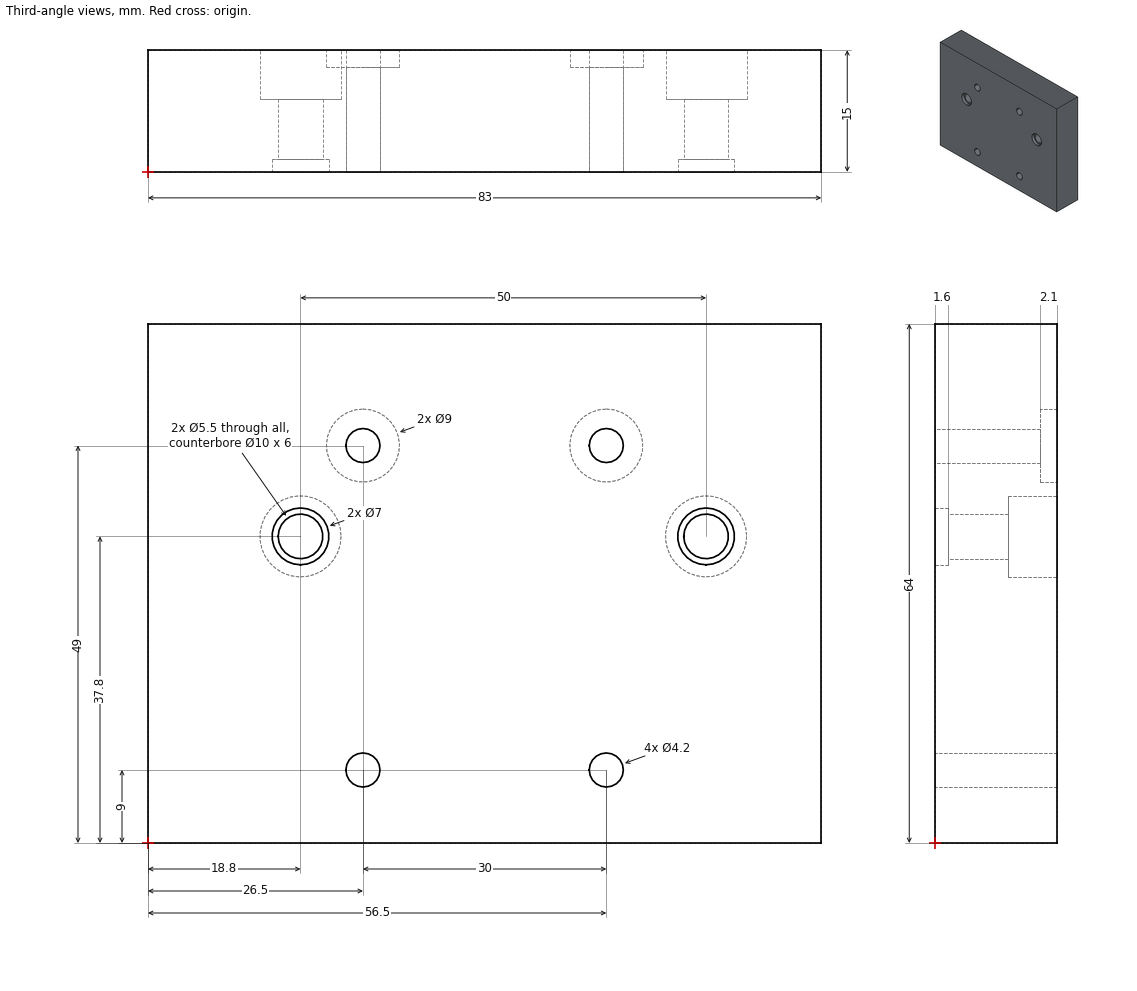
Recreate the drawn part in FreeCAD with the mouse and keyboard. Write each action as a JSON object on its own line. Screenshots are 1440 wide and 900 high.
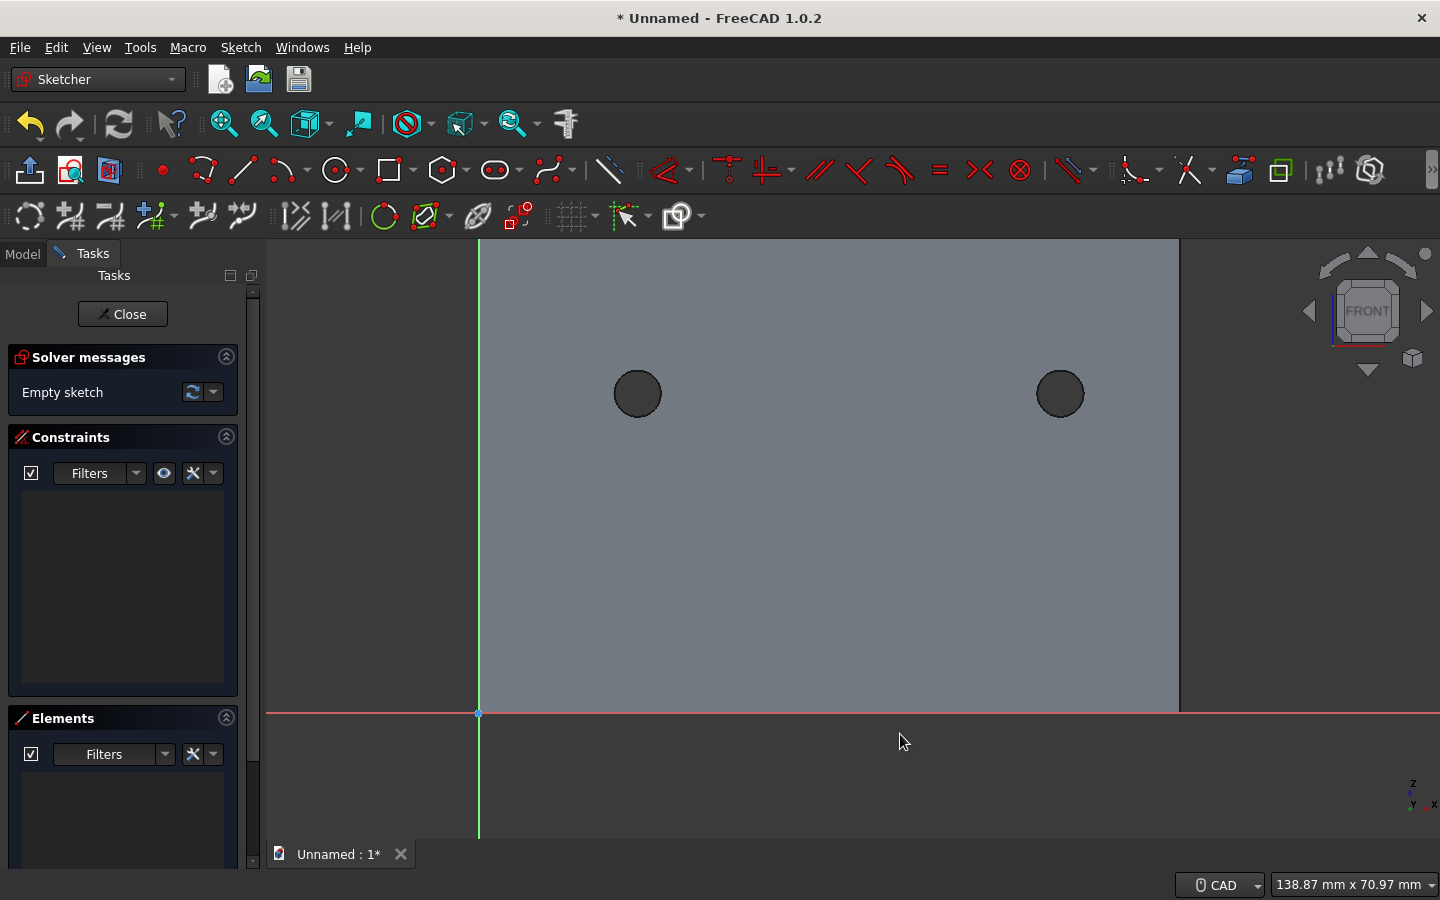
{"action": "left_click", "coordinate": [336, 170]}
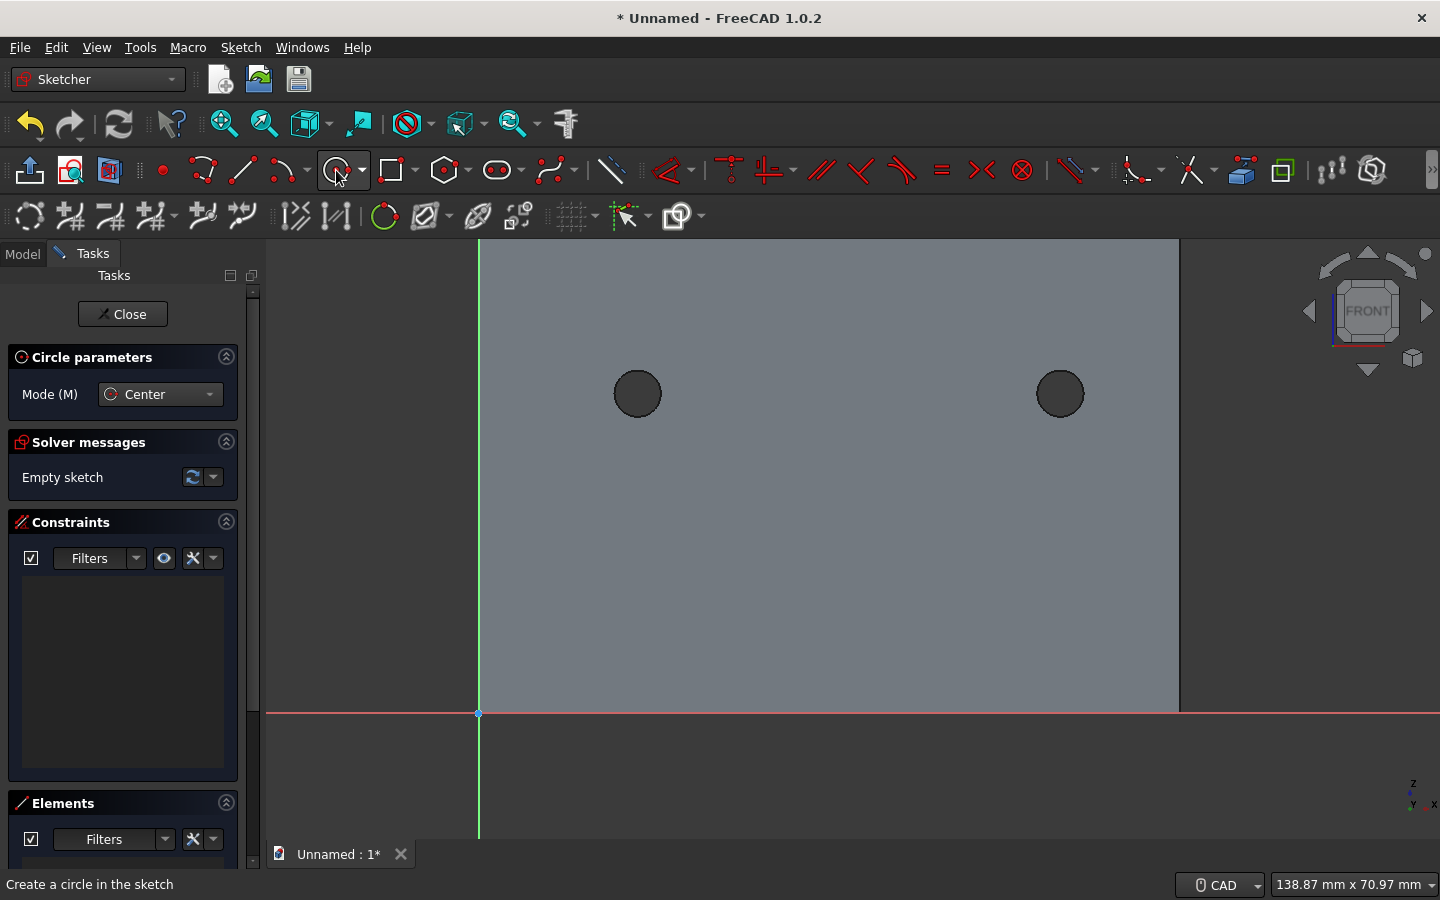
{"action": "left_click", "coordinate": [638, 394]}
{"action": "left_click", "coordinate": [659, 373]}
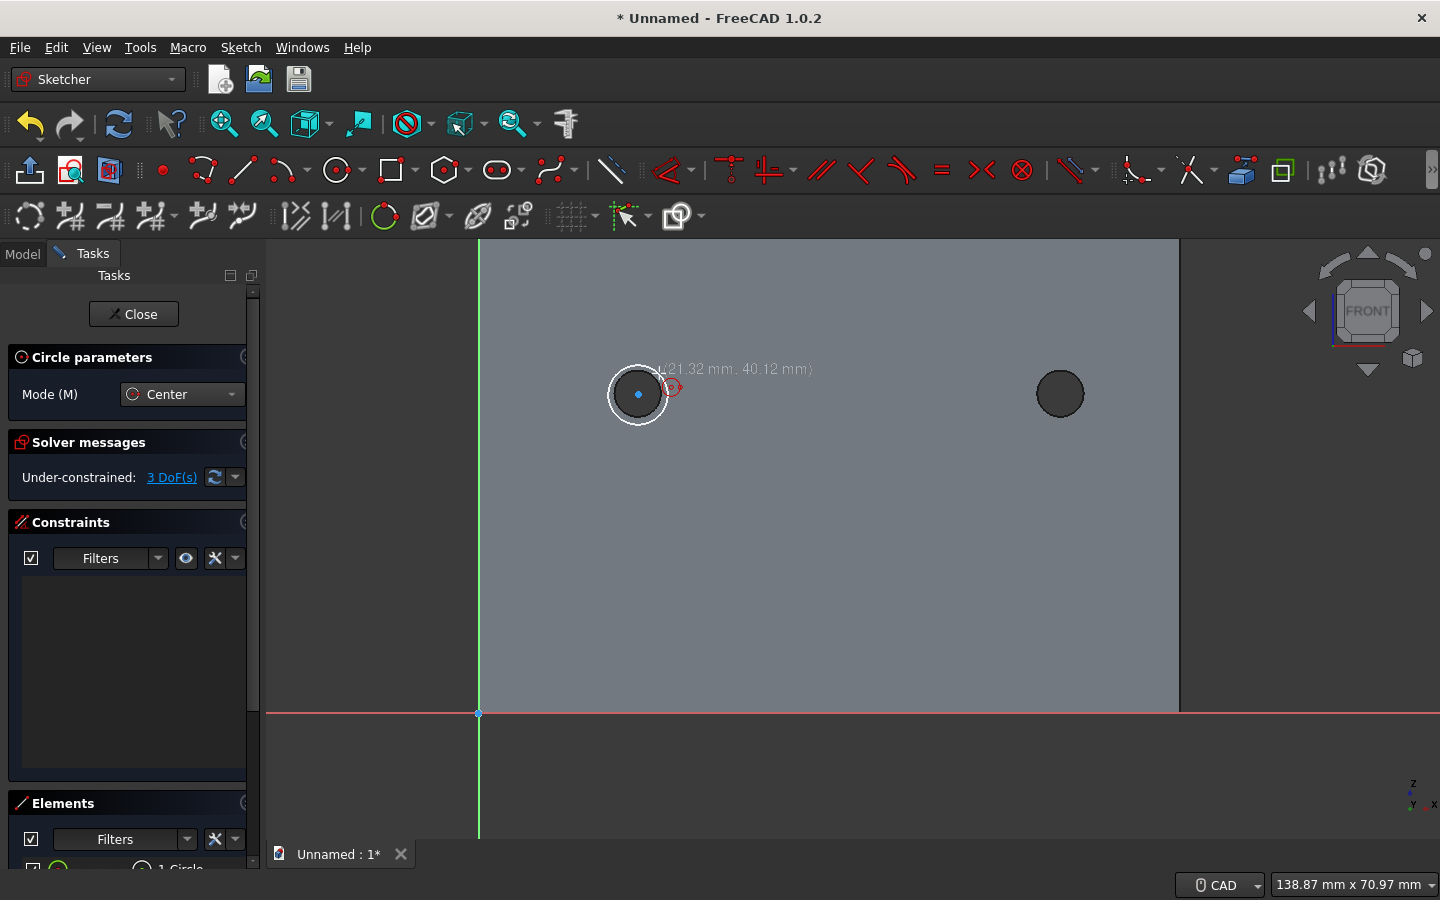
{"action": "left_click", "coordinate": [1060, 394]}
{"action": "left_click", "coordinate": [1081, 373]}
{"action": "key", "text": "Escape"}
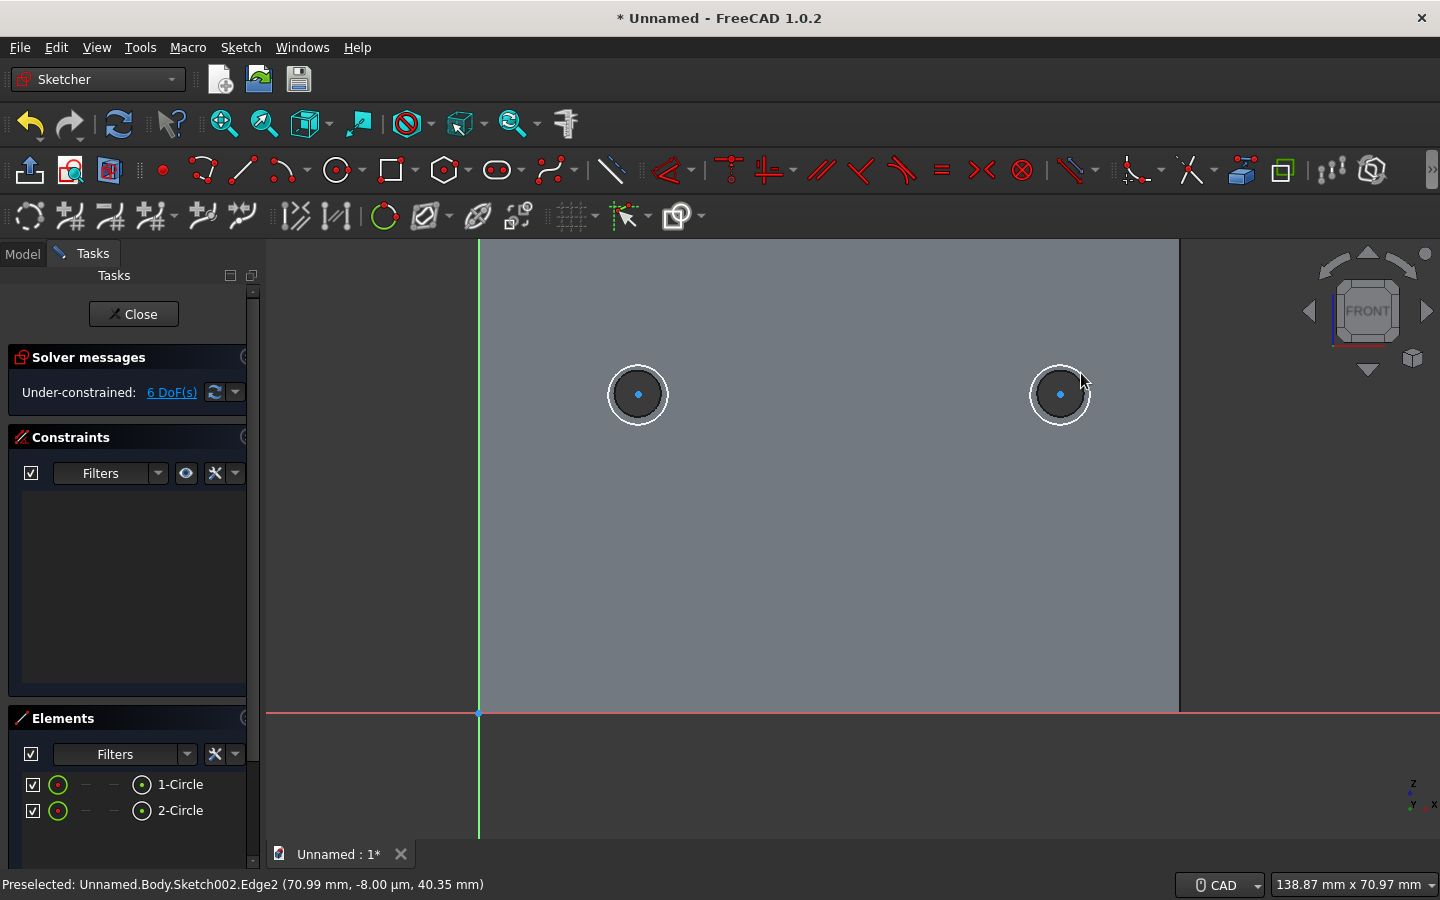
{"action": "left_click", "coordinate": [659, 374]}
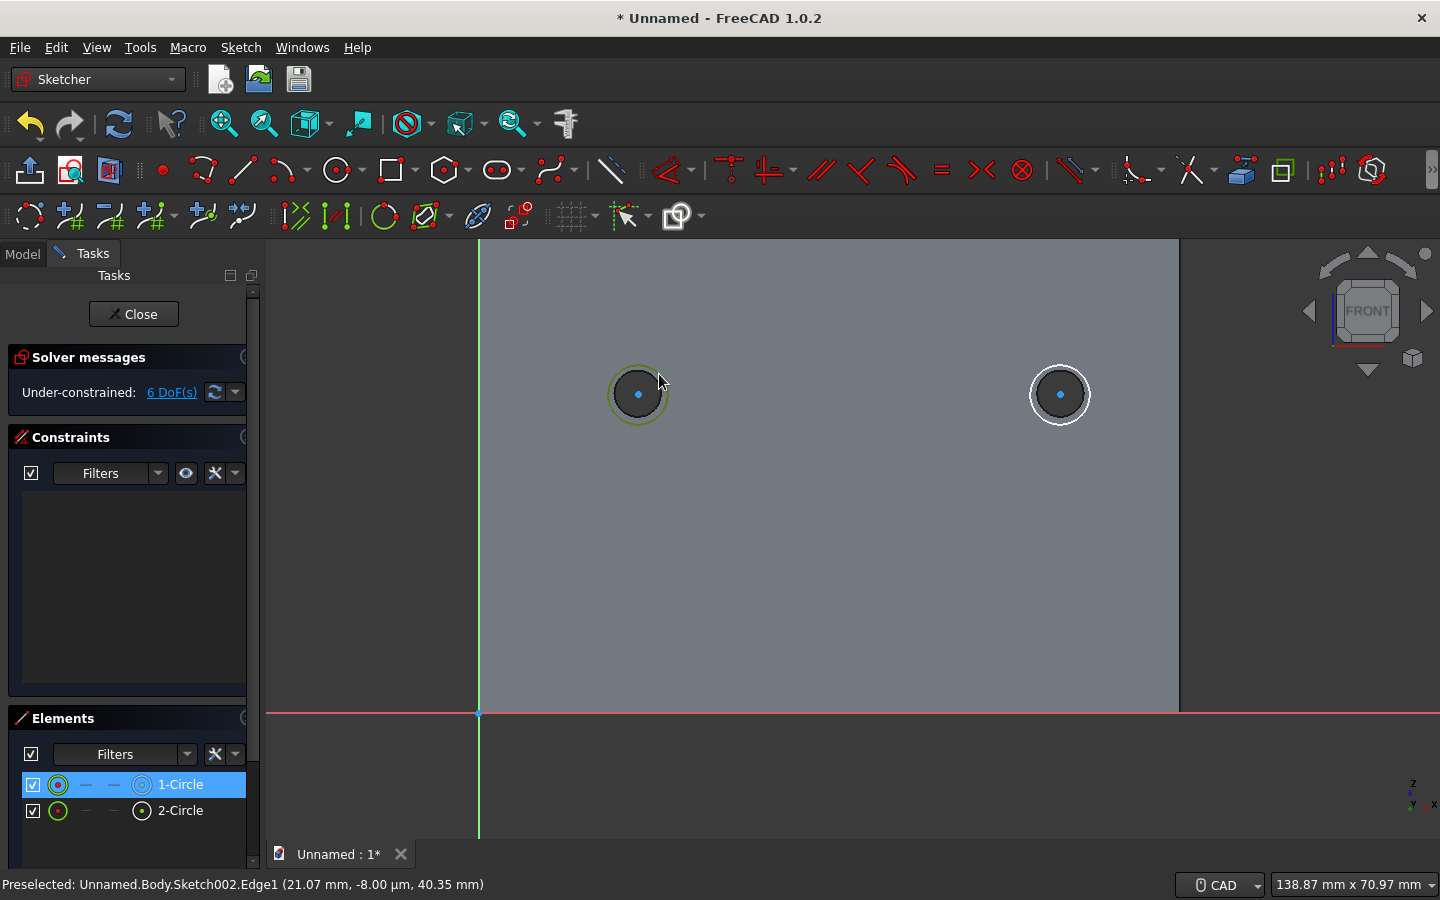
{"action": "left_click", "coordinate": [1081, 374]}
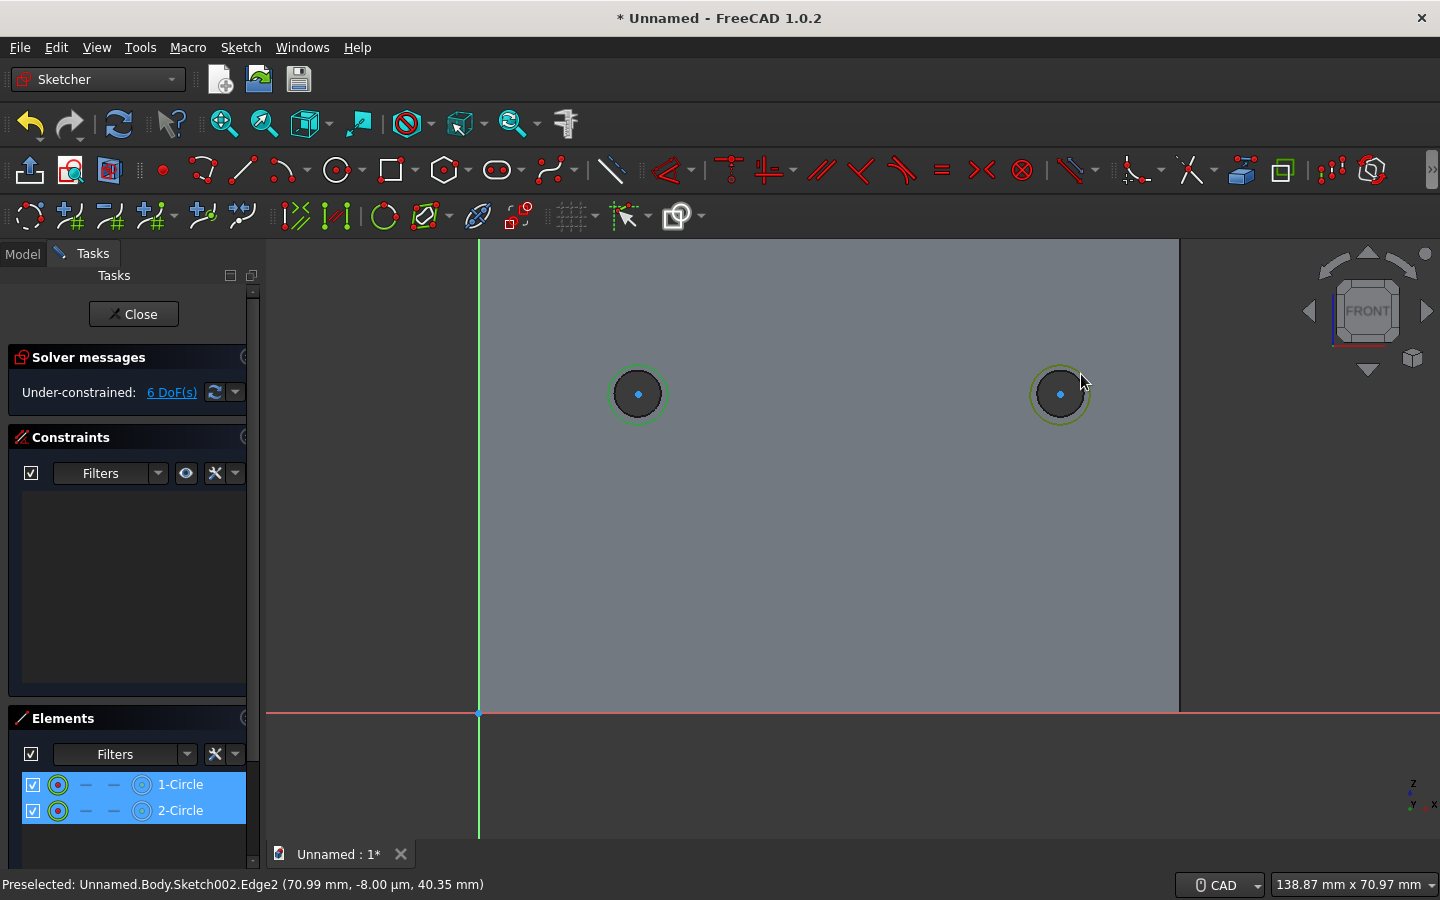
{"action": "left_click", "coordinate": [942, 170]}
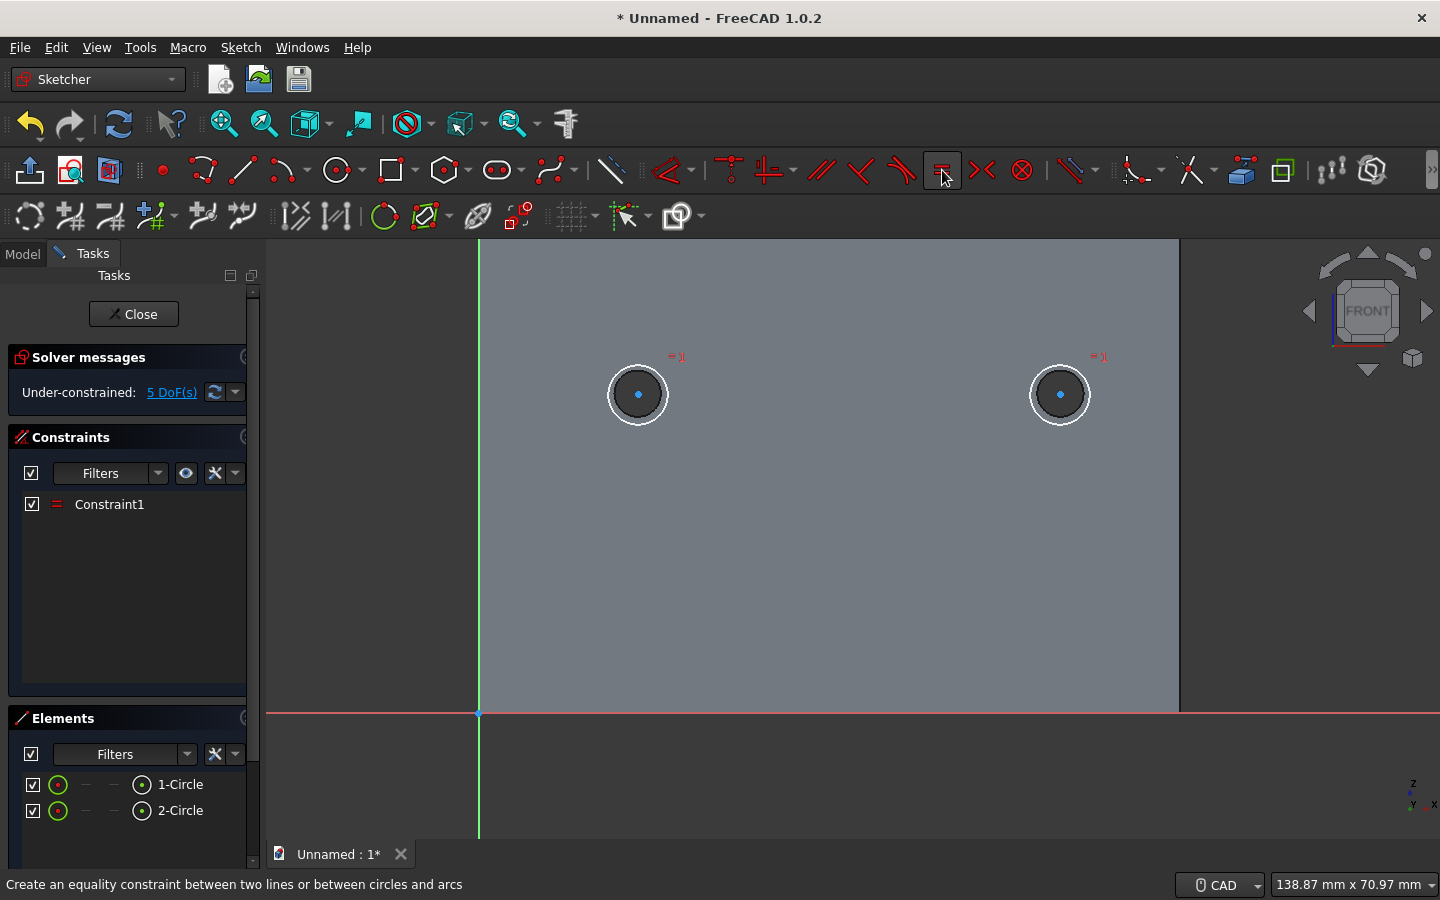
{"action": "left_click", "coordinate": [666, 170]}